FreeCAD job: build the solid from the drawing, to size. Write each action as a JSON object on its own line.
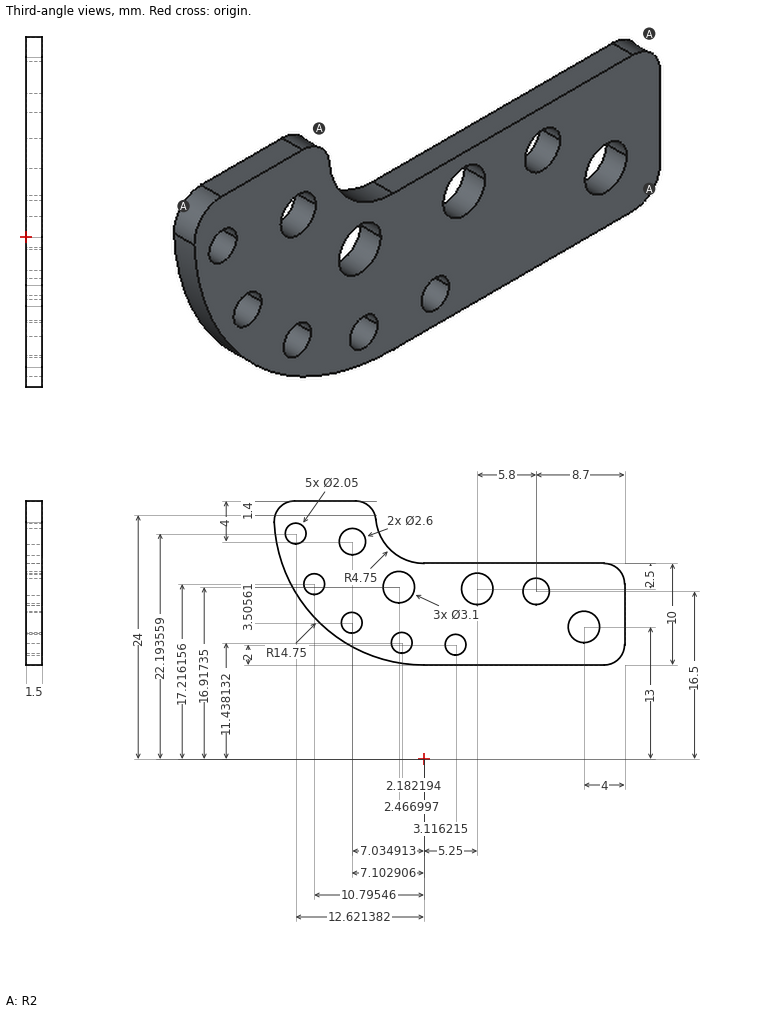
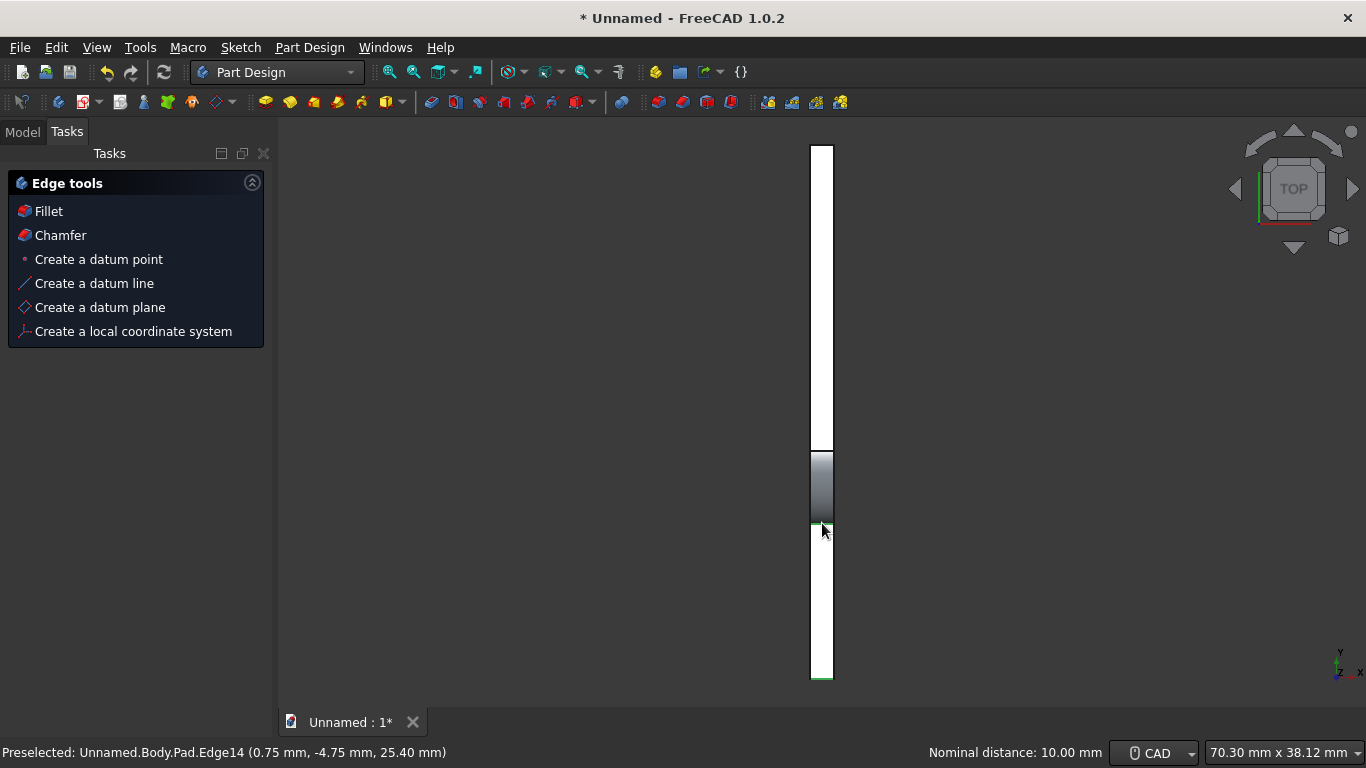
{"action": "key", "text": "1"}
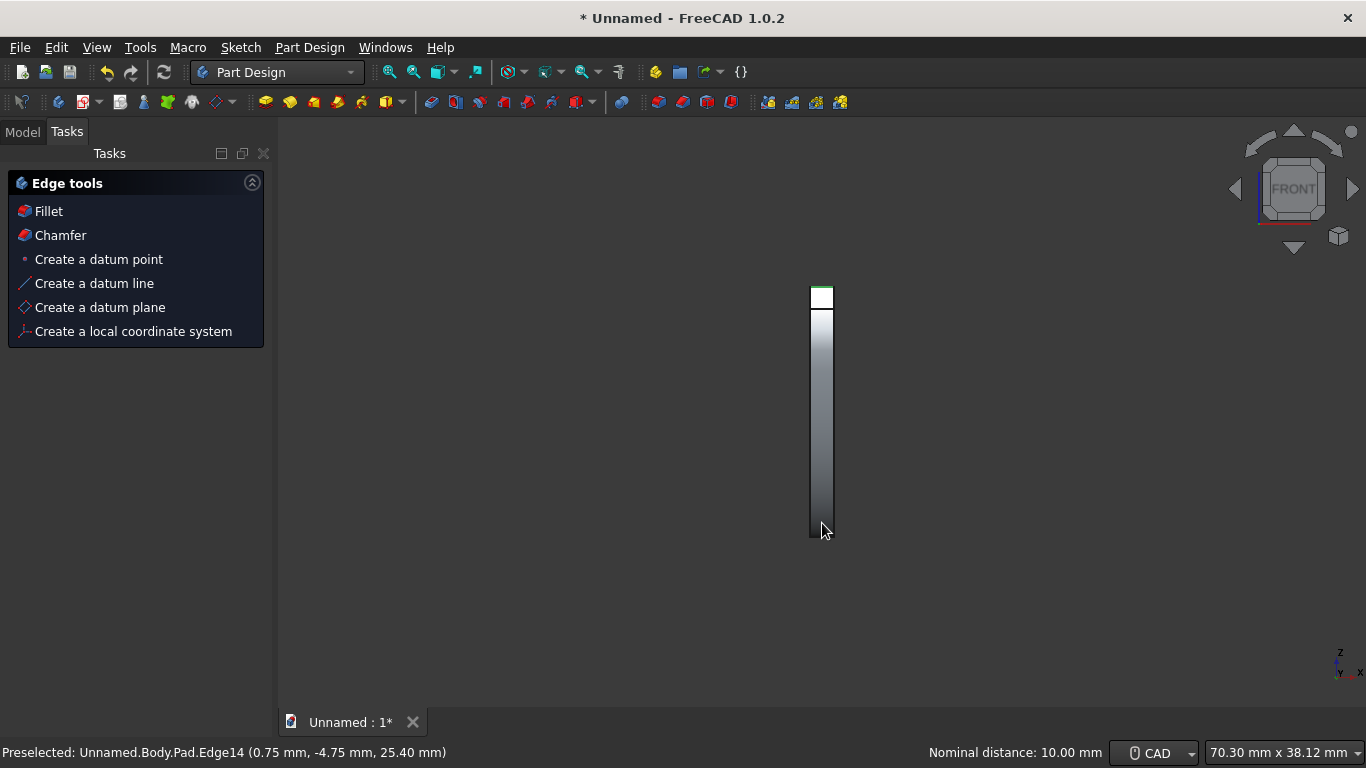
{"action": "key", "text": "v f"}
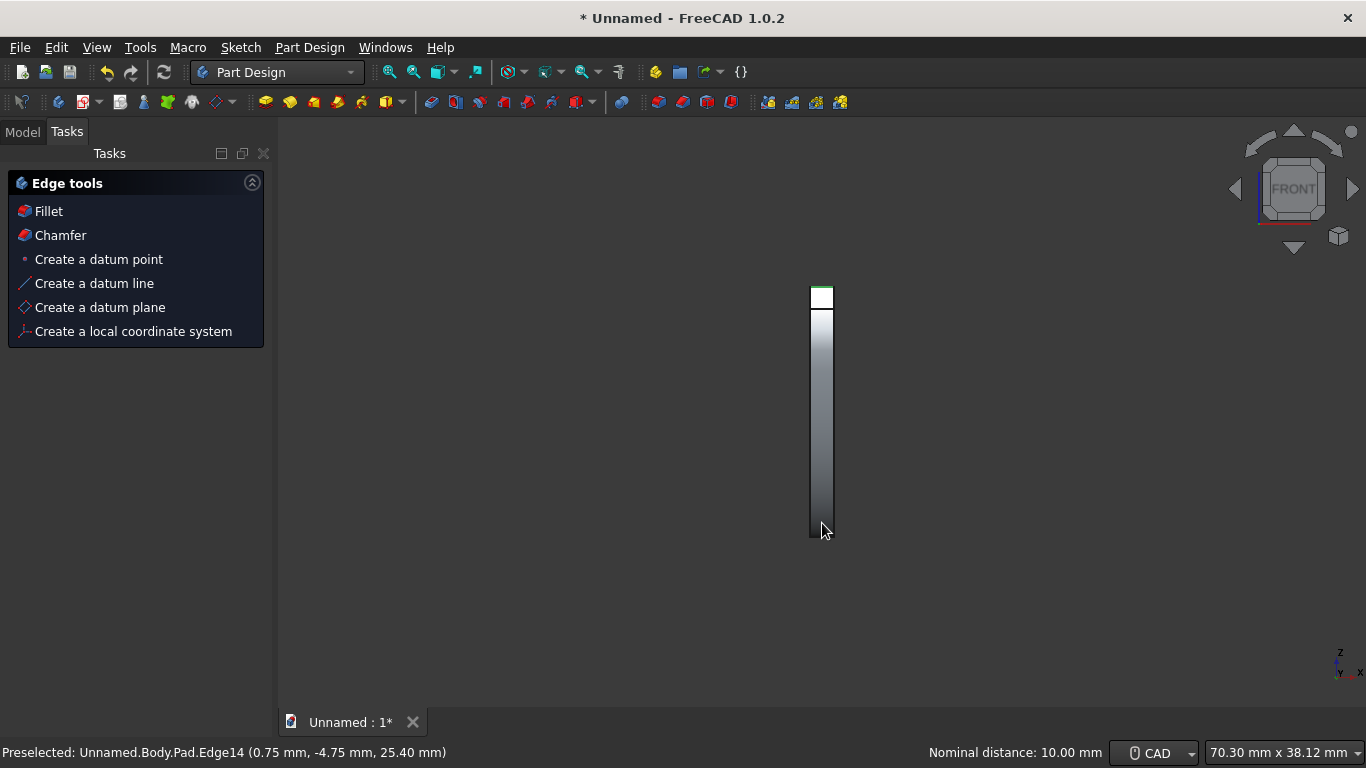
{"action": "key", "text": "3"}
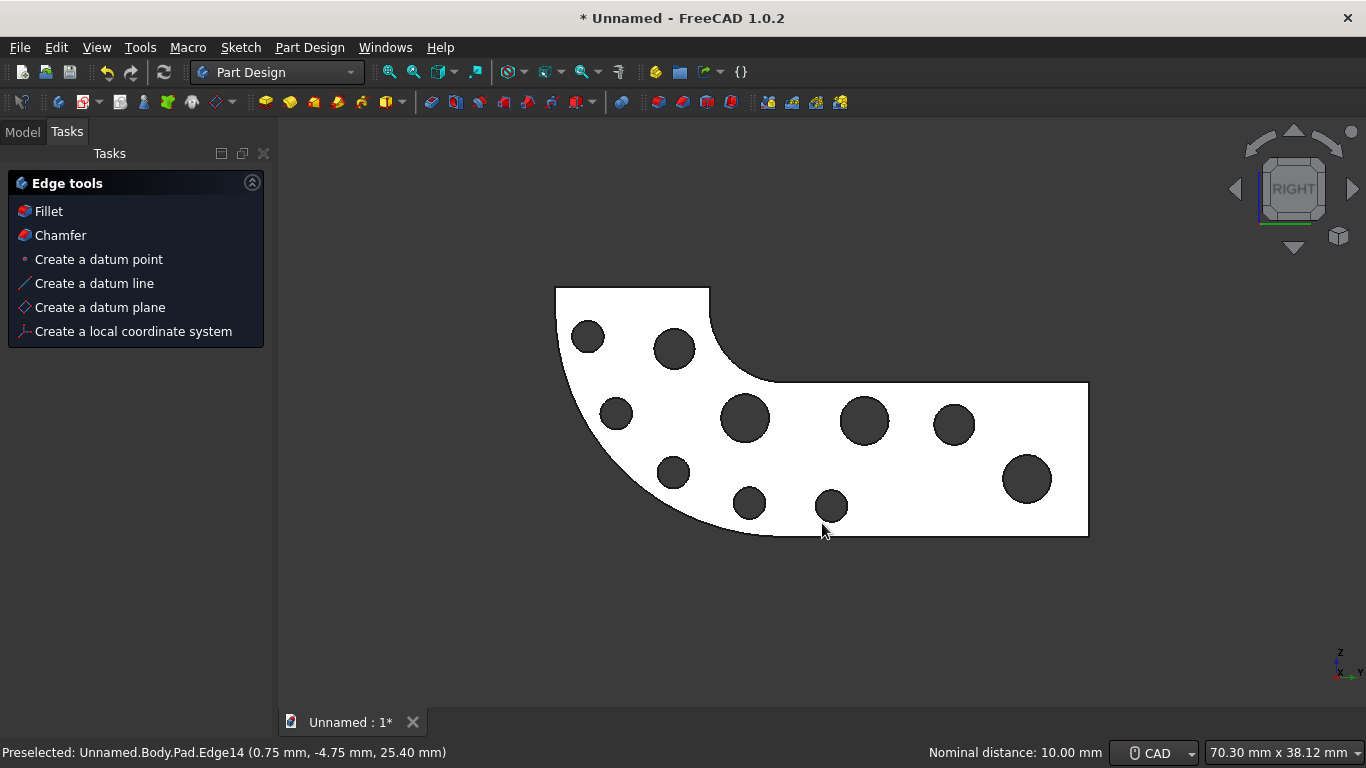
{"action": "key", "text": "5"}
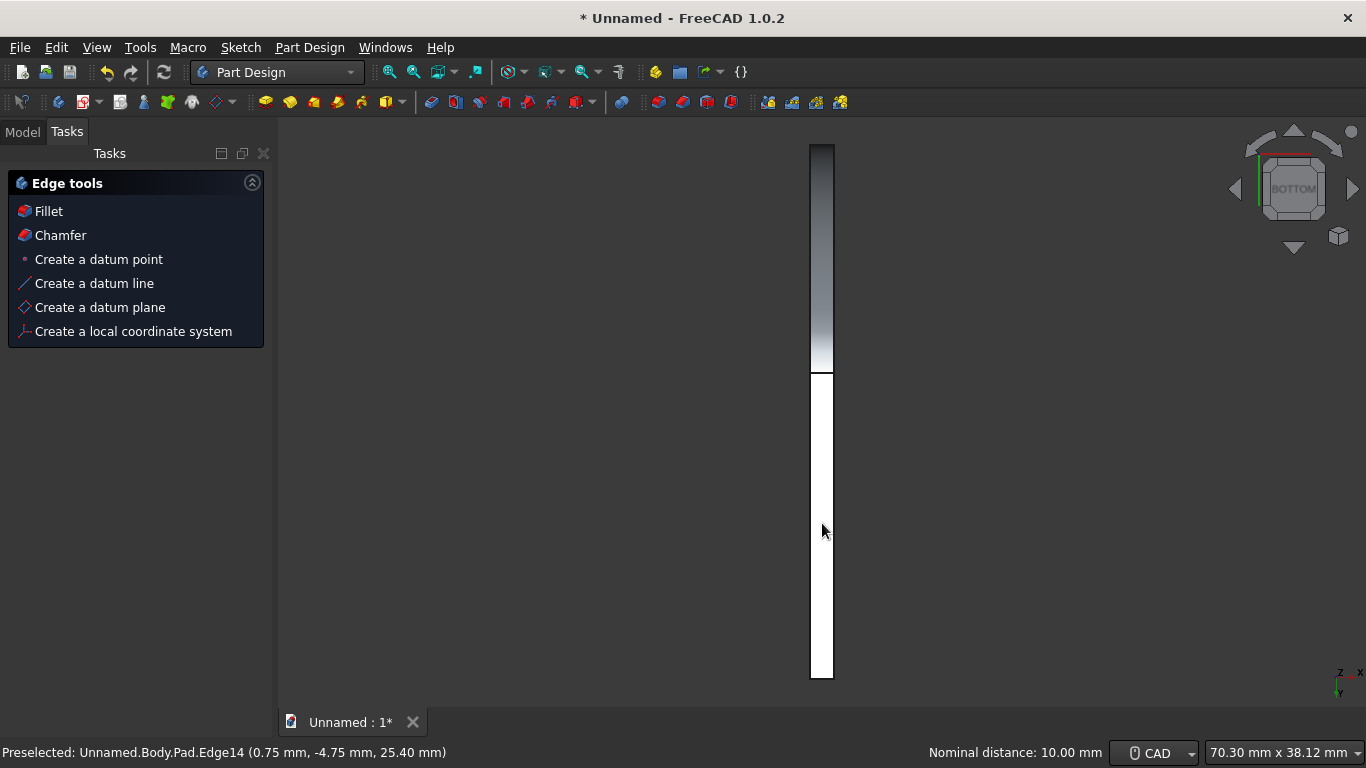
{"action": "left_click", "coordinate": [822, 678], "text": "ctrl"}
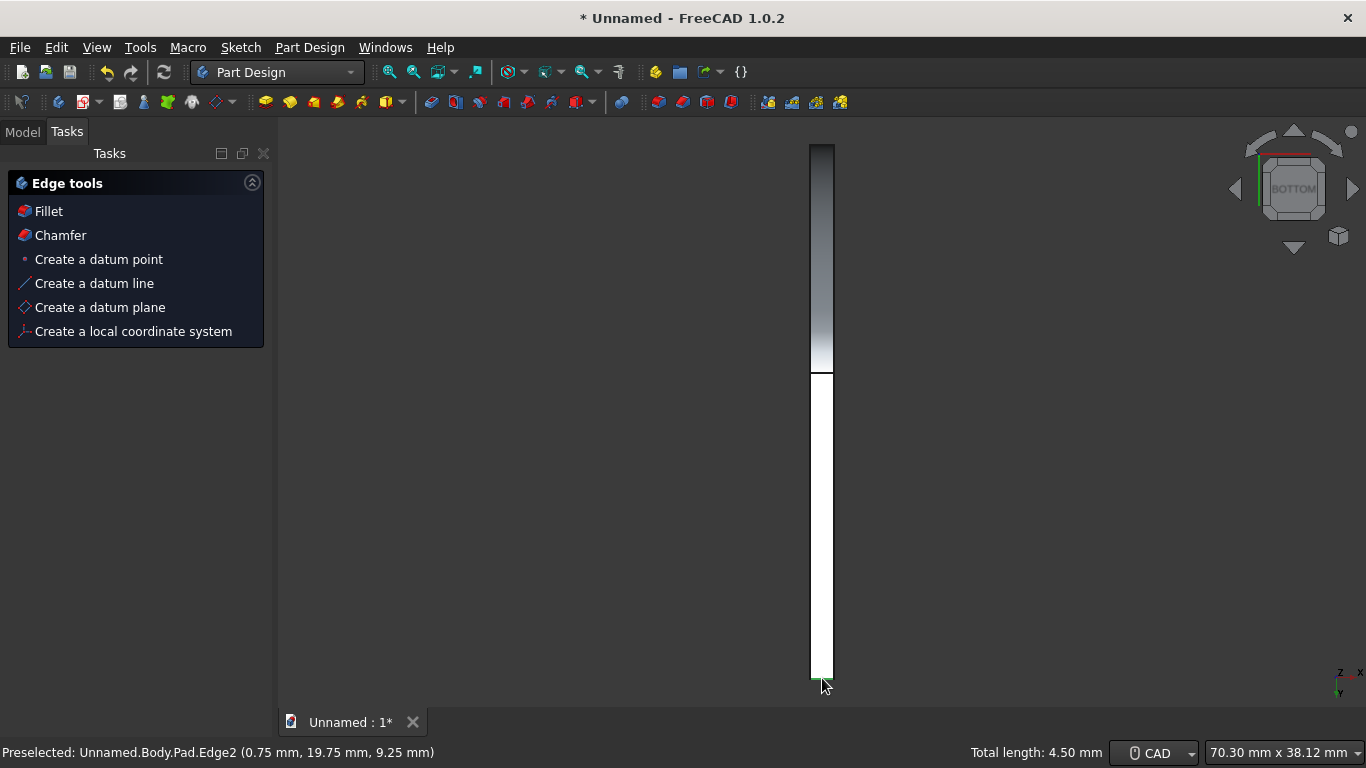
{"action": "key", "text": "4"}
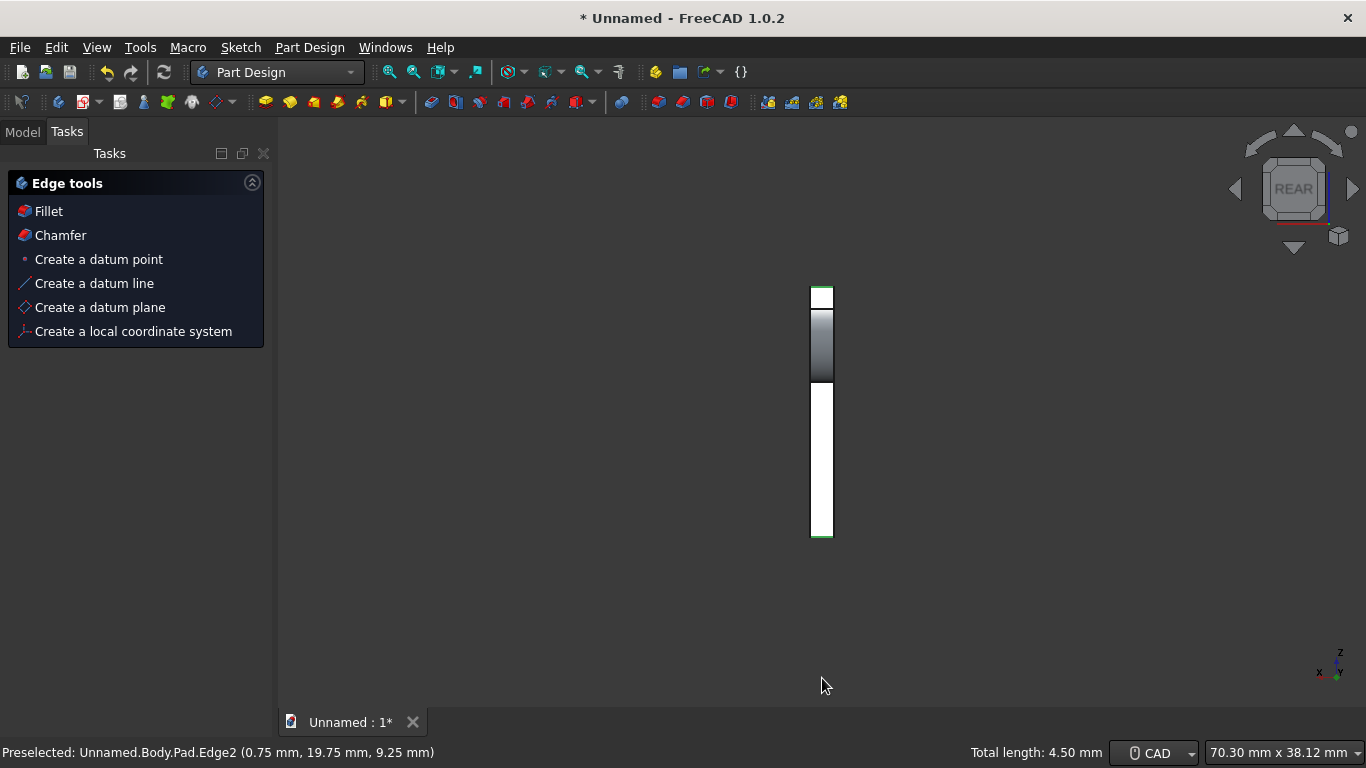
{"action": "left_click", "coordinate": [390, 72]}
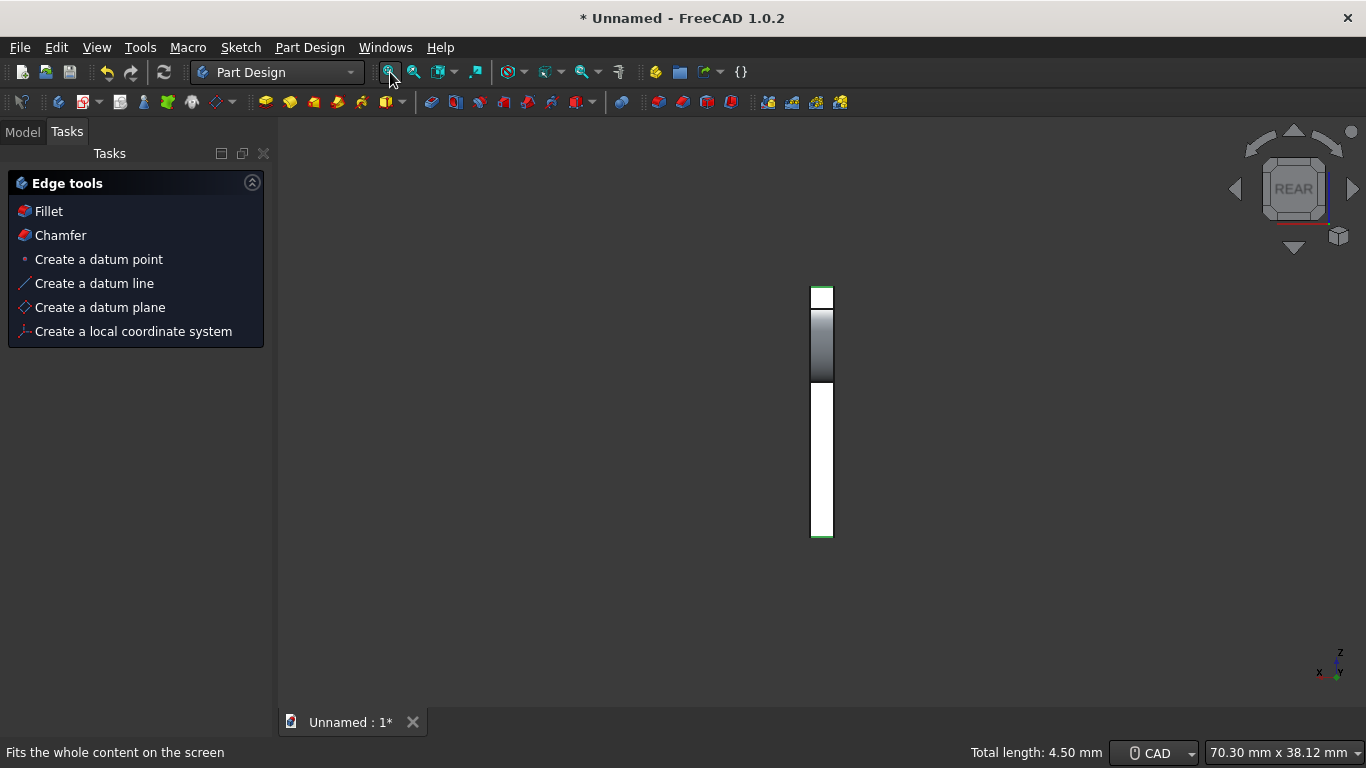
{"action": "left_click", "coordinate": [822, 381], "text": "ctrl"}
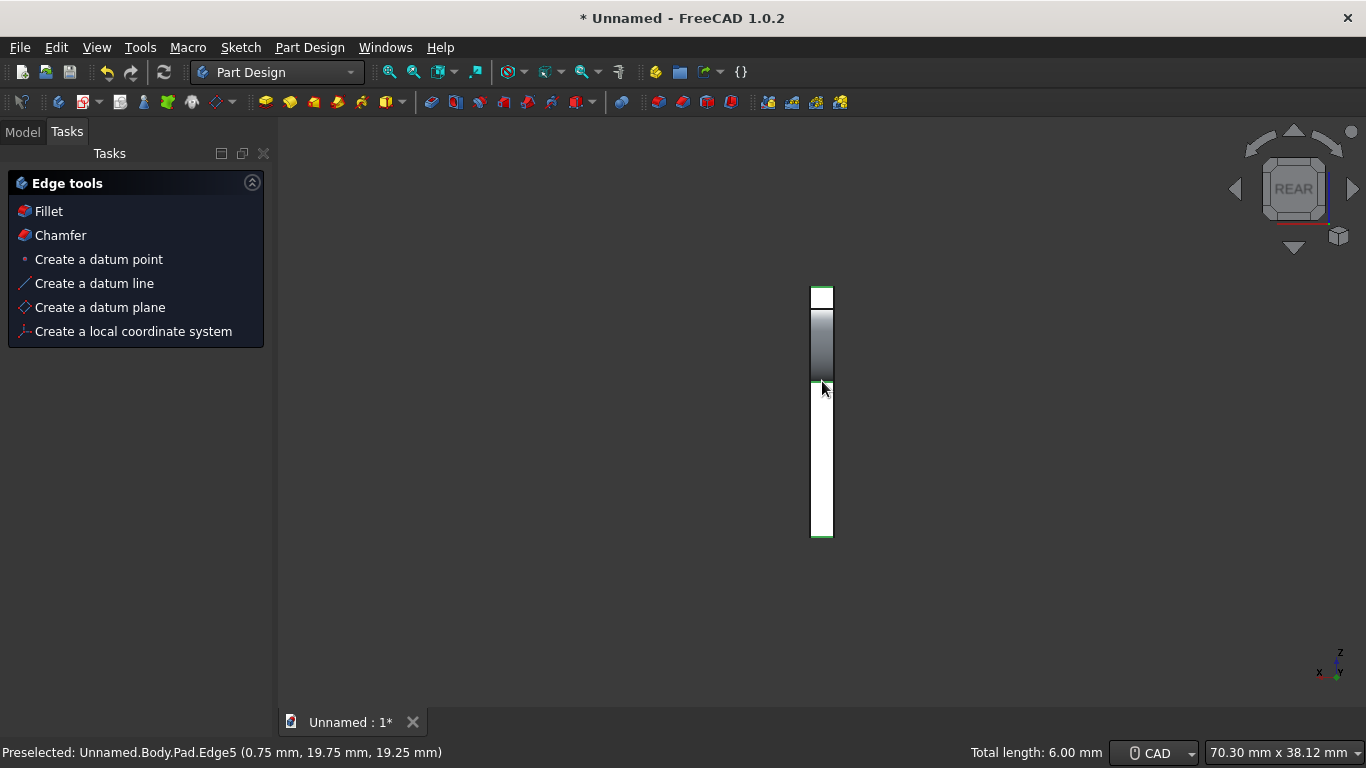
{"action": "left_click", "coordinate": [660, 102]}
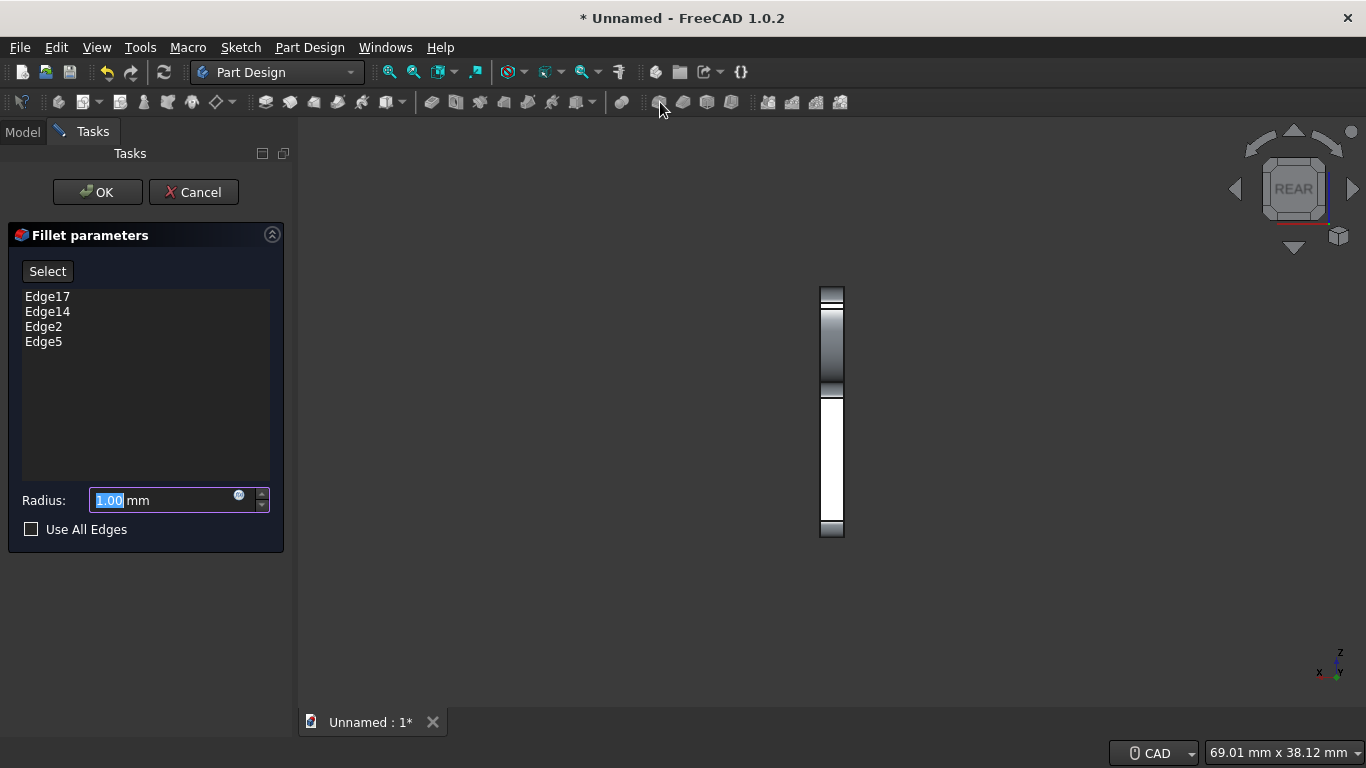
{"action": "type", "text": "2"}
{"action": "key", "text": "Tab"}